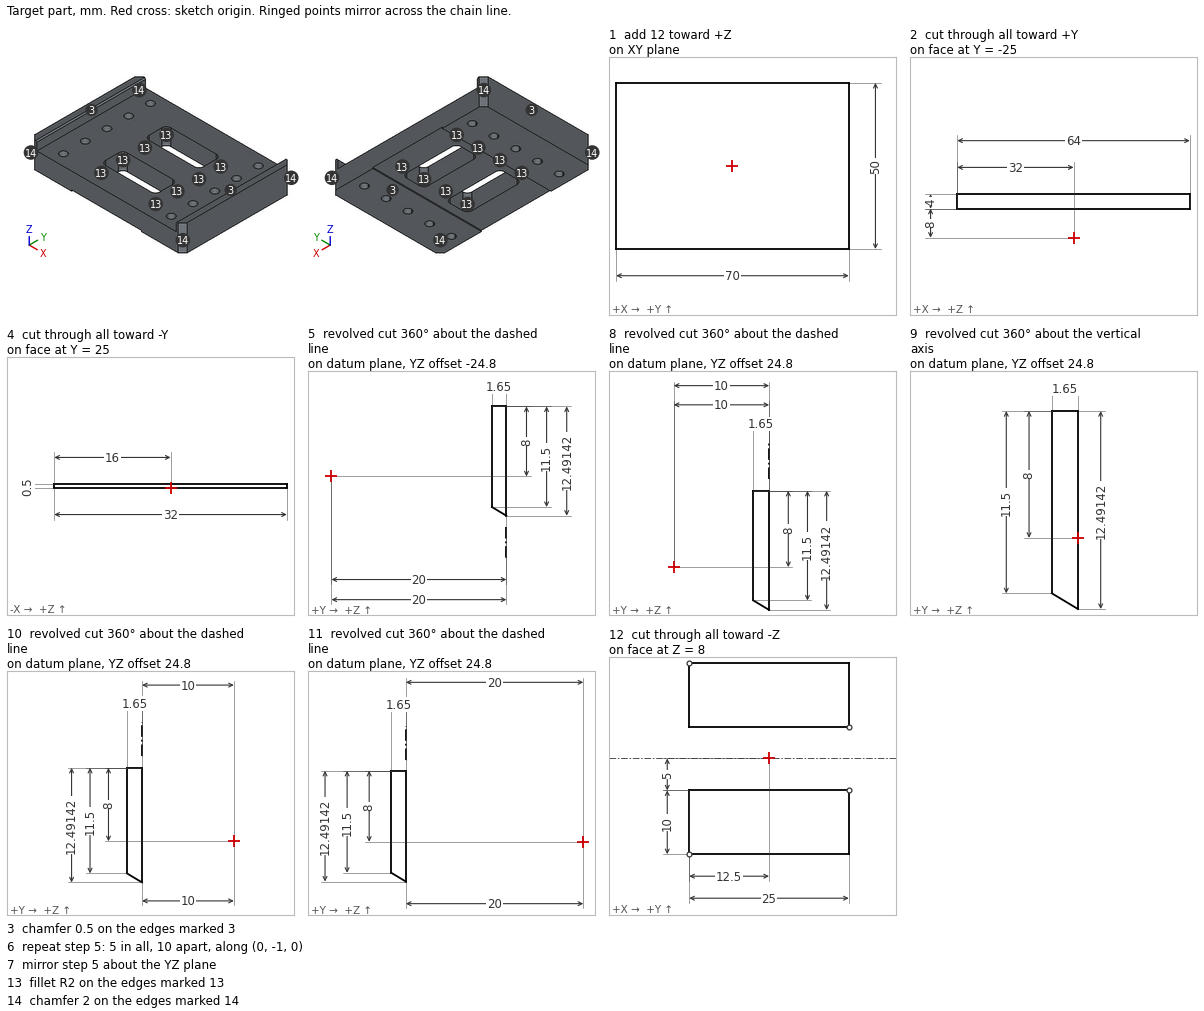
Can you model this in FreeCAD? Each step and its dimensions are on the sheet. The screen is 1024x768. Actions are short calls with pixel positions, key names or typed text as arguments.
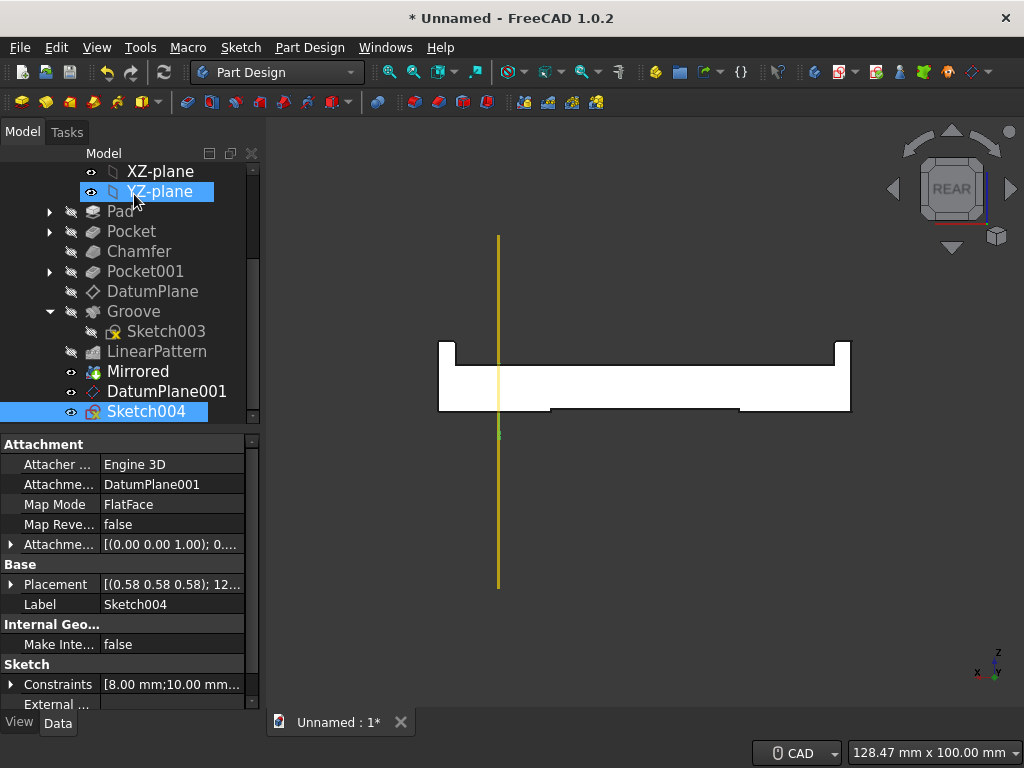
click(236, 102)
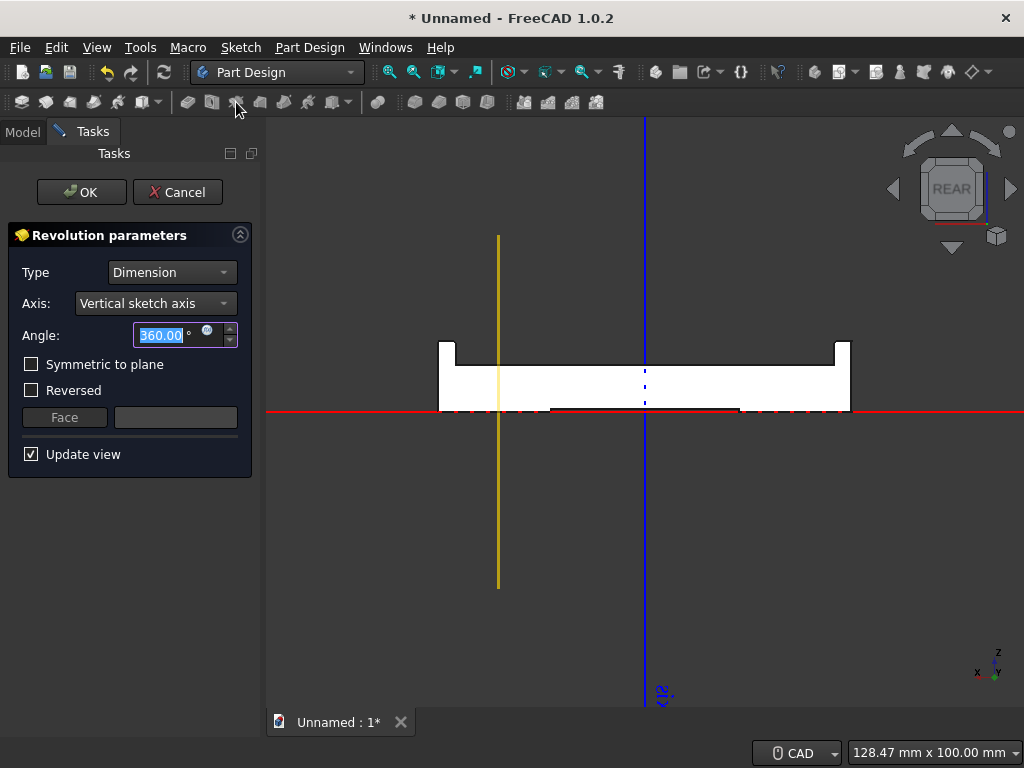
click(156, 304)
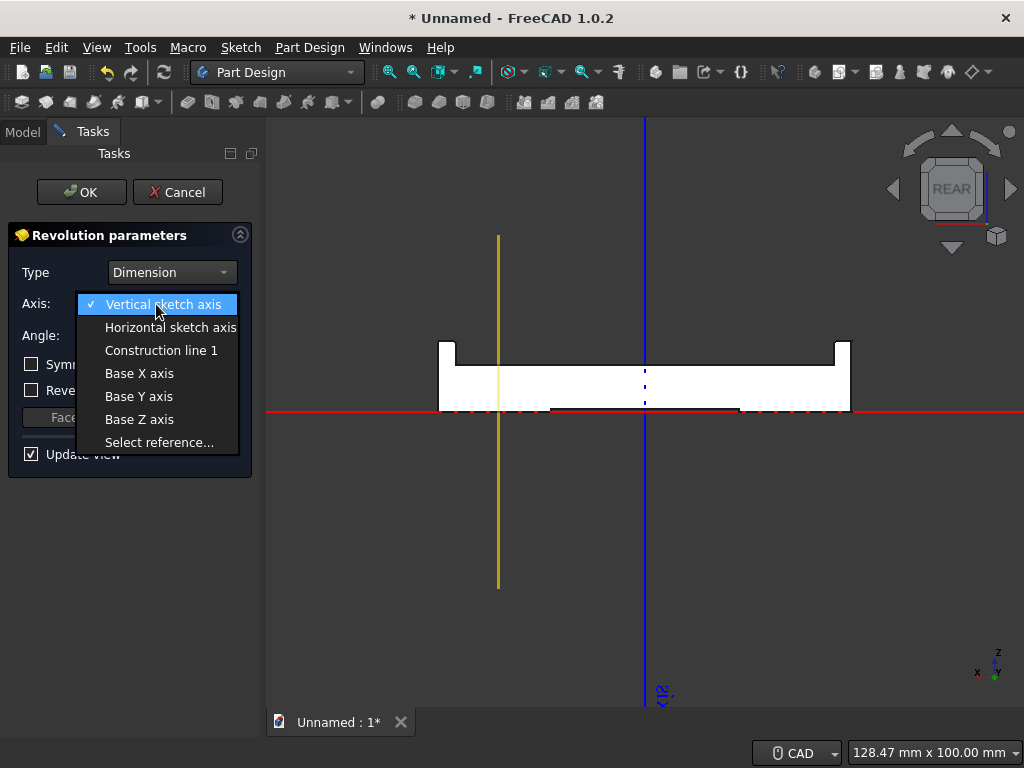
click(156, 350)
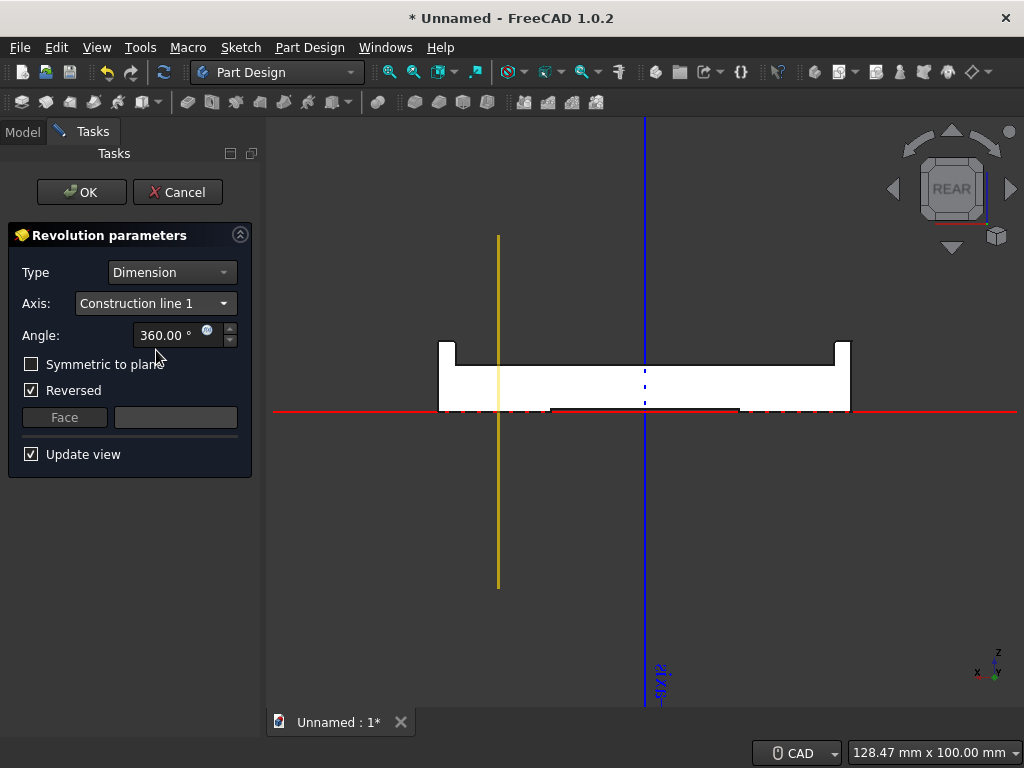
click(82, 192)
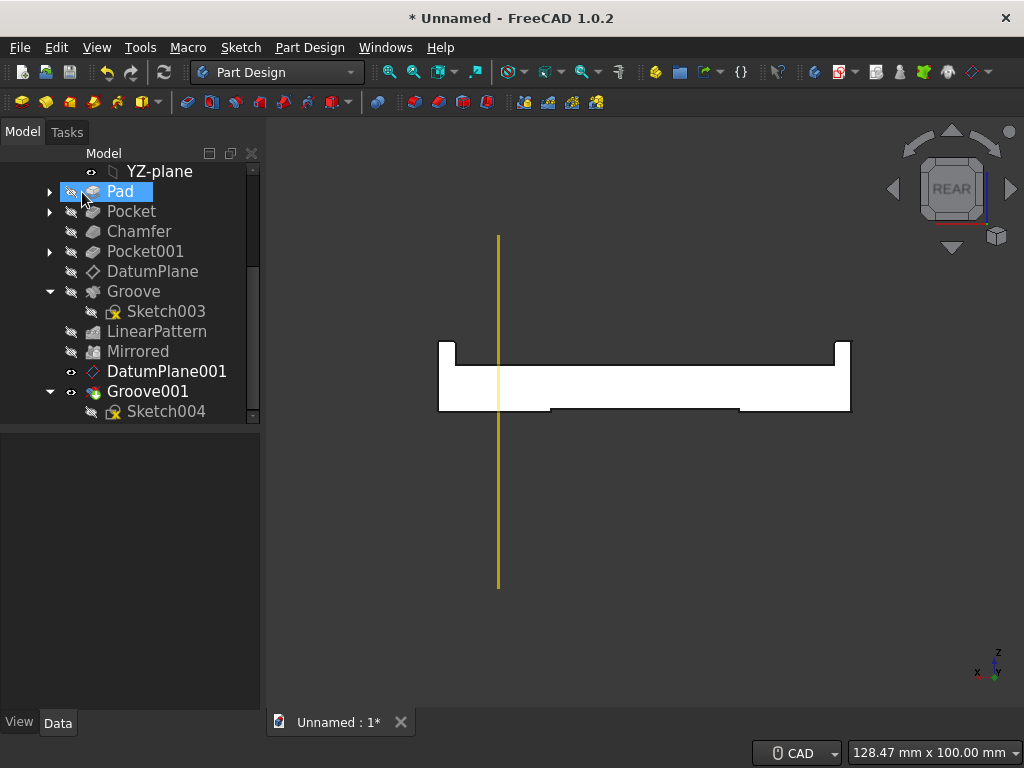
click(116, 372)
key(space)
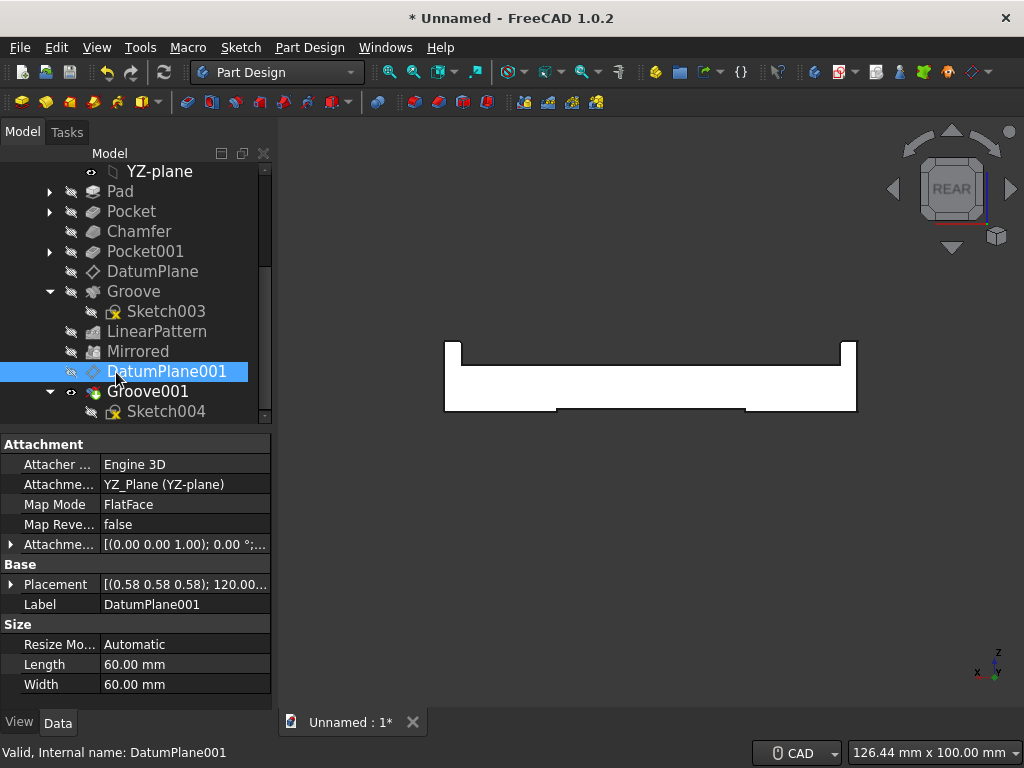
scroll(160, 287, down, 3)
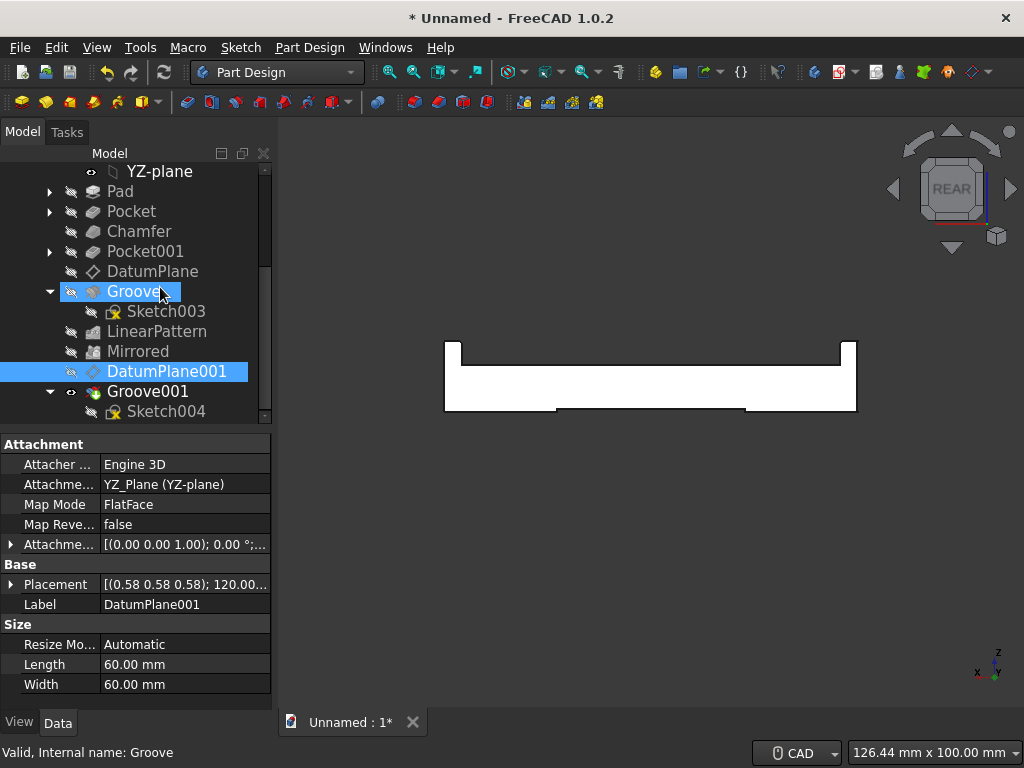
scroll(160, 287, up, 15)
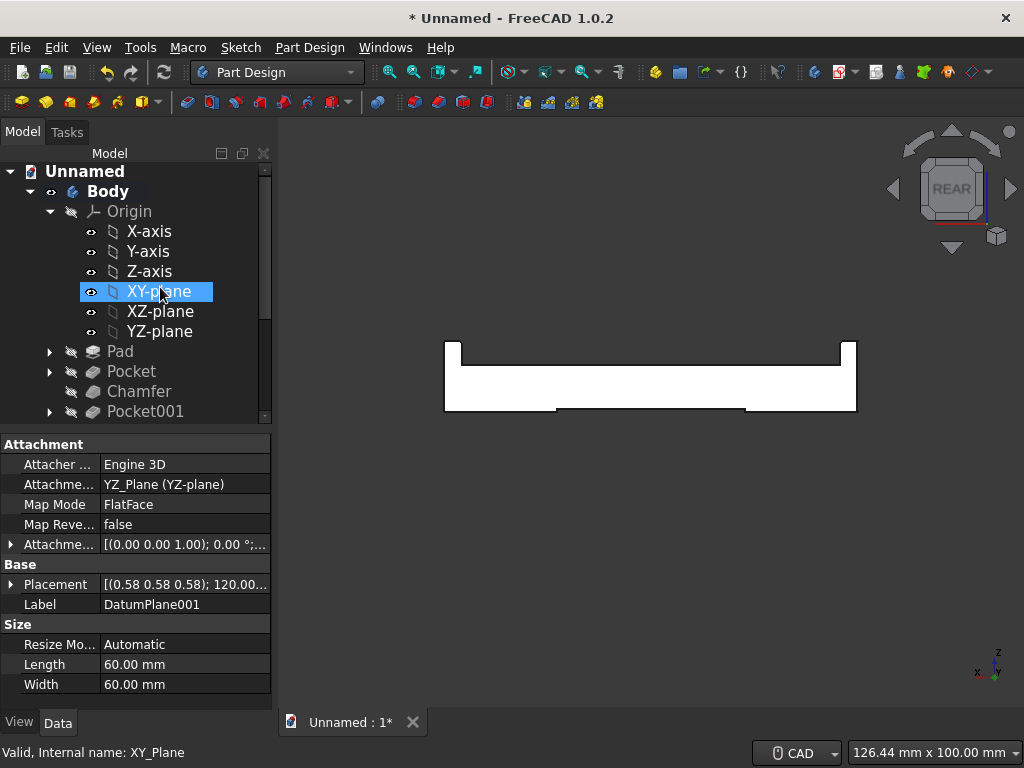
click(136, 332)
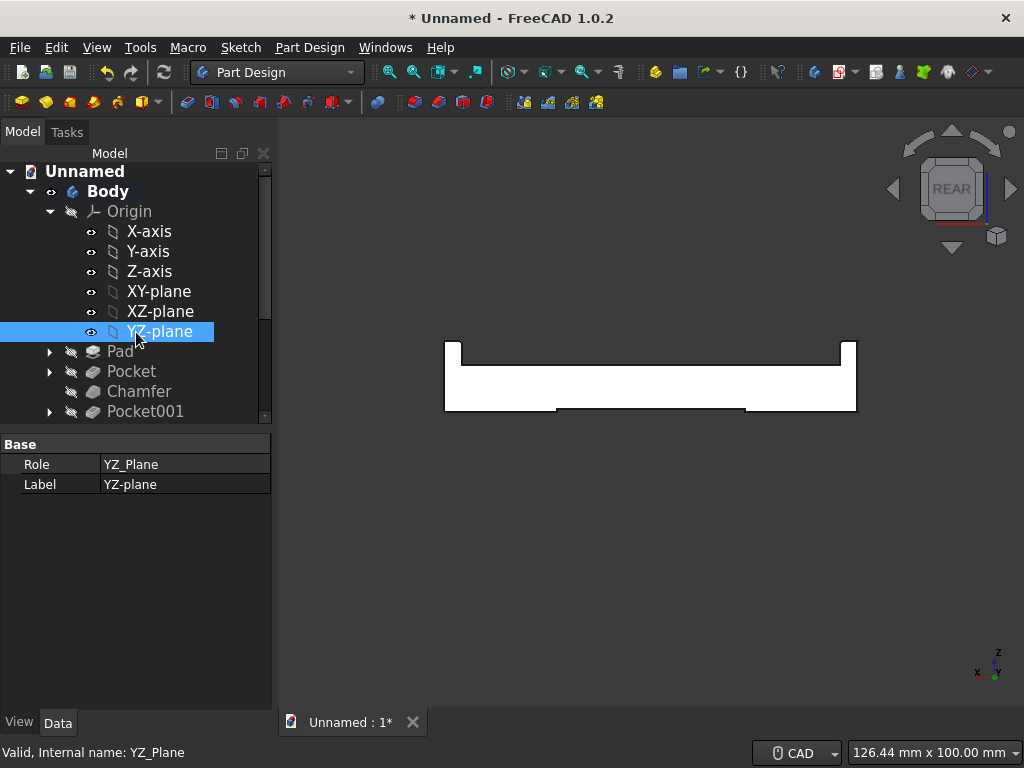
click(972, 72)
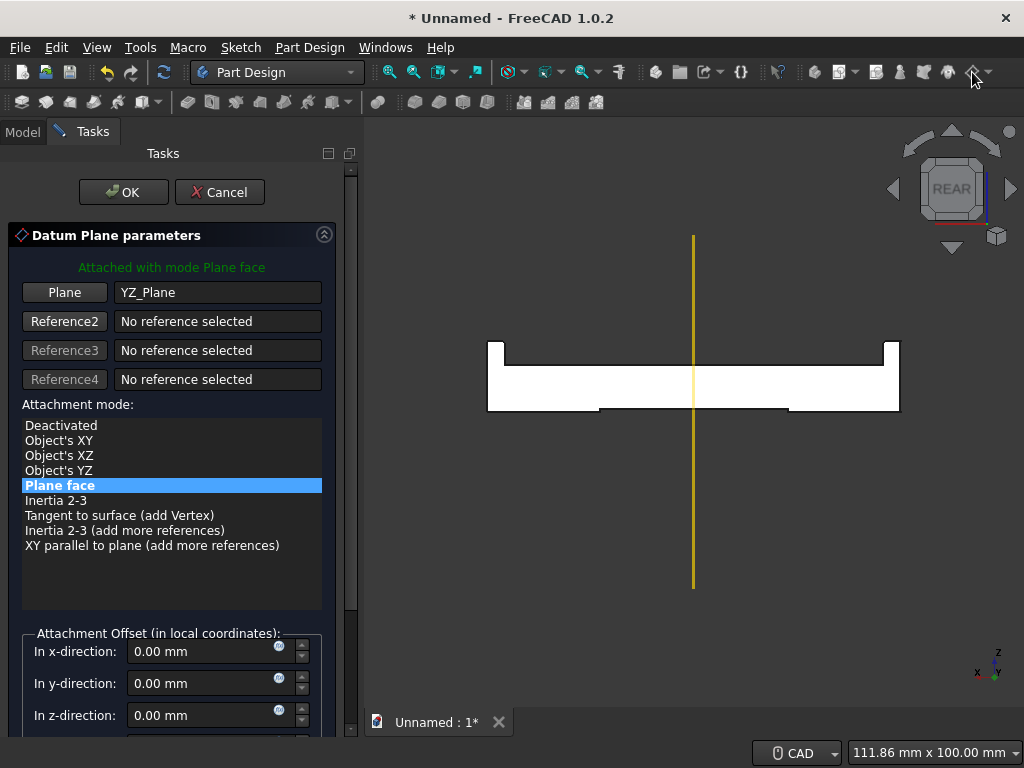
triple_click(210, 715)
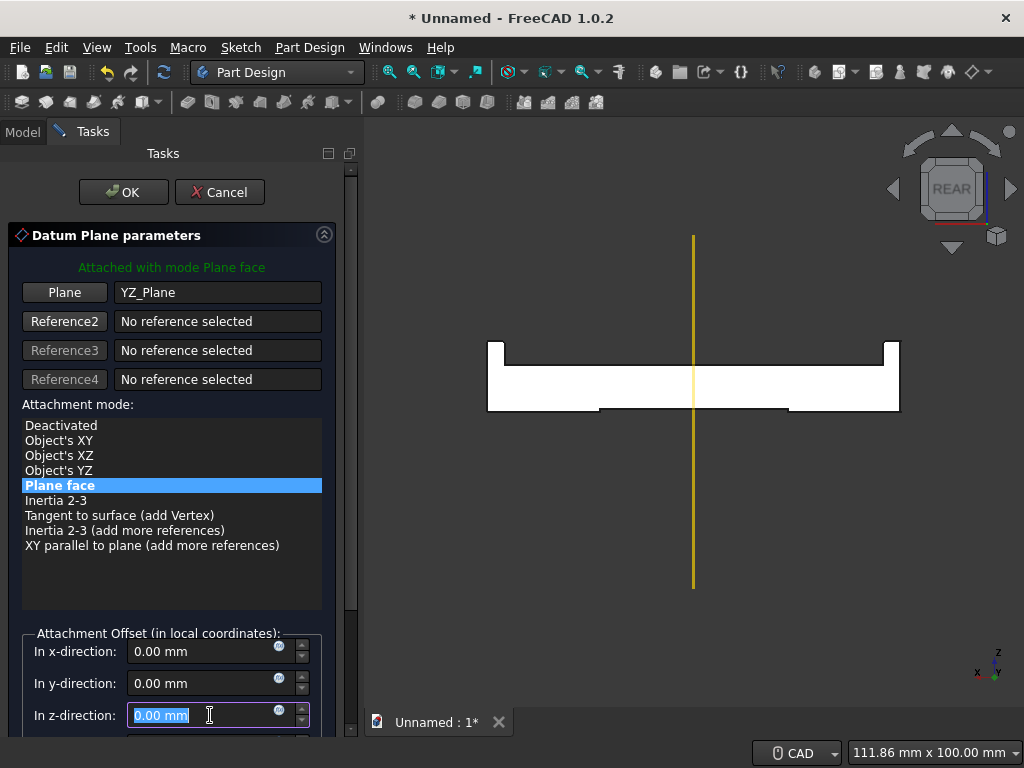
text(24.8)
key(Tab)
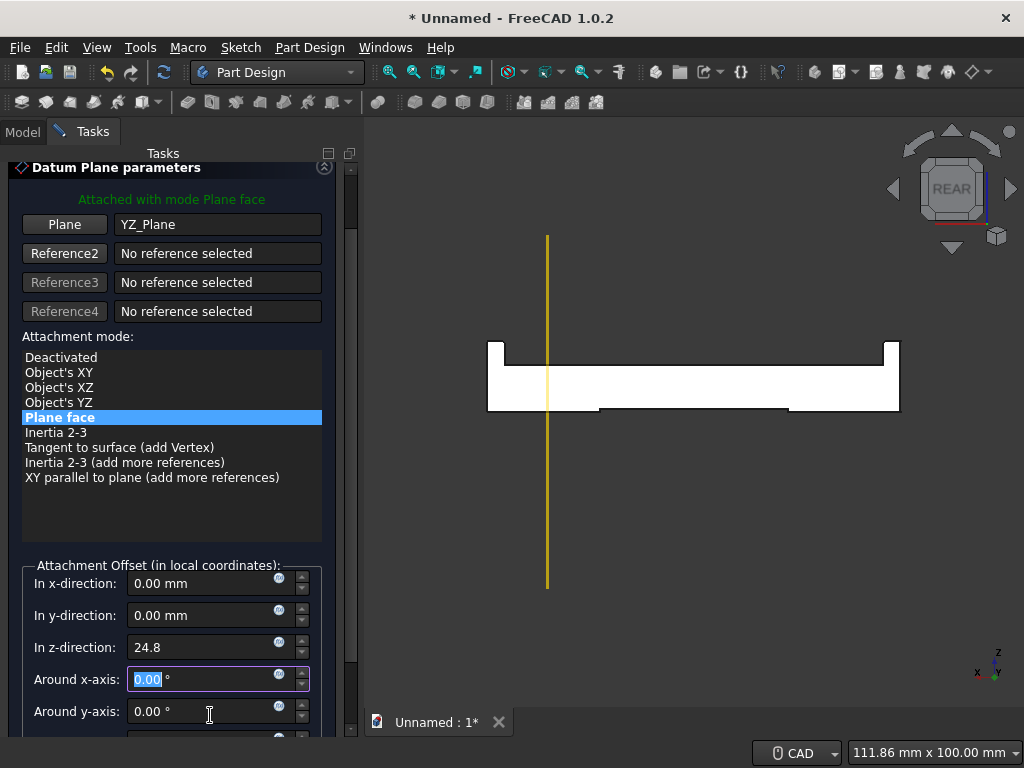
scroll(351, 450, up, 2)